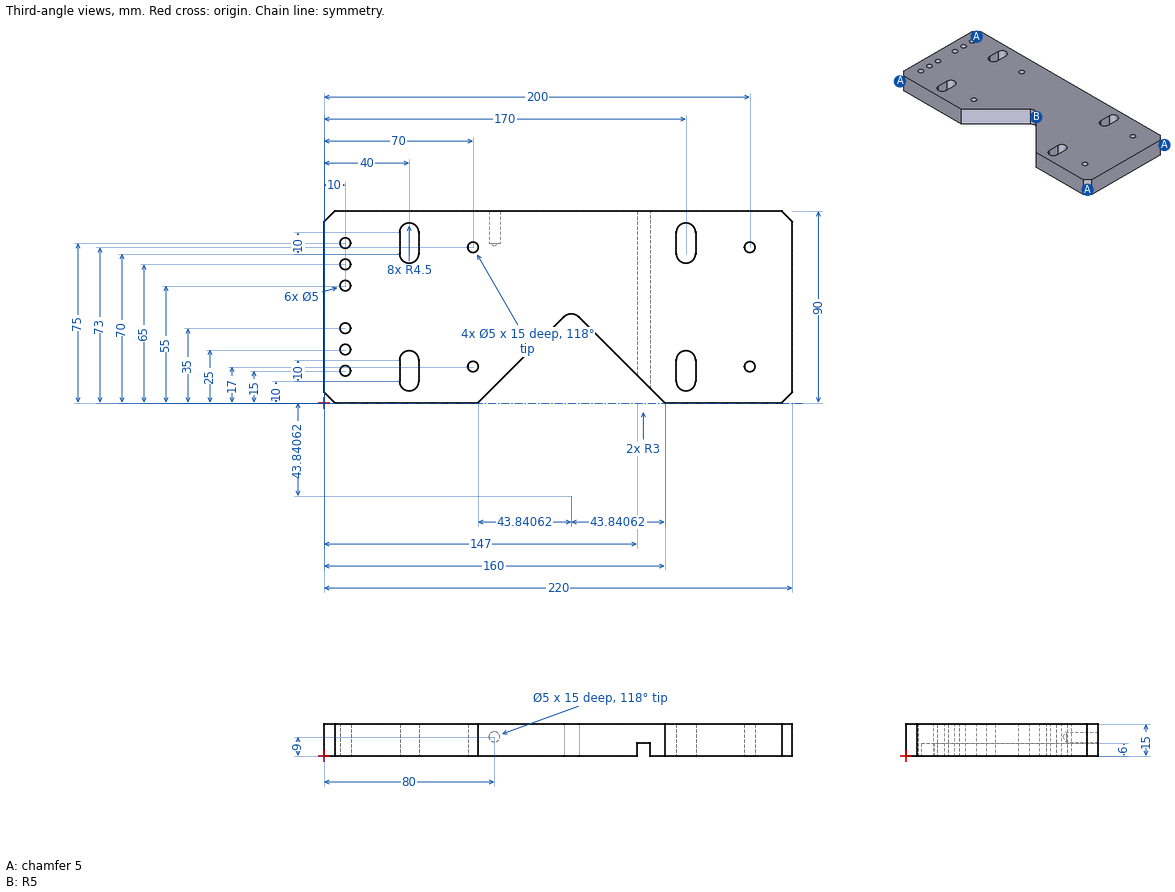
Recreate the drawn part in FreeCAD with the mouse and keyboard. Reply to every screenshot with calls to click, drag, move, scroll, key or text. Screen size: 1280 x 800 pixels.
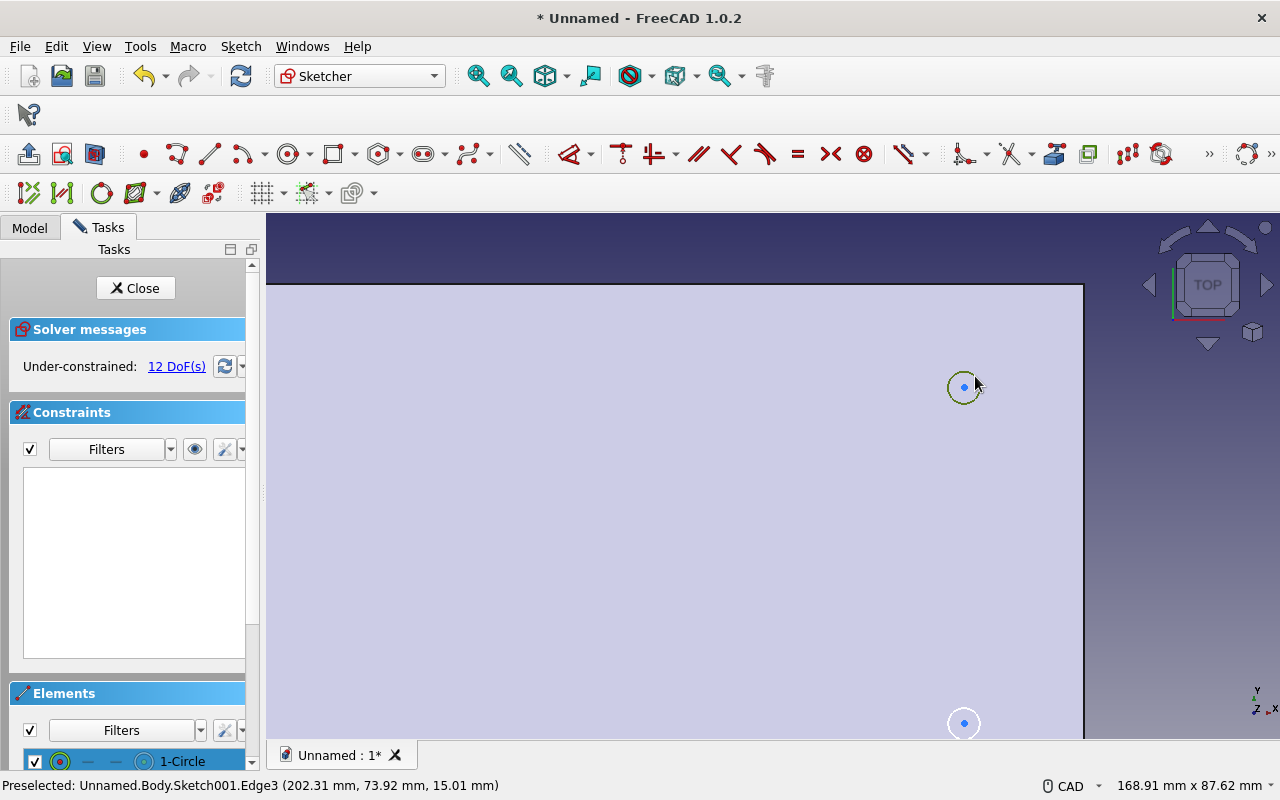
click(964, 708)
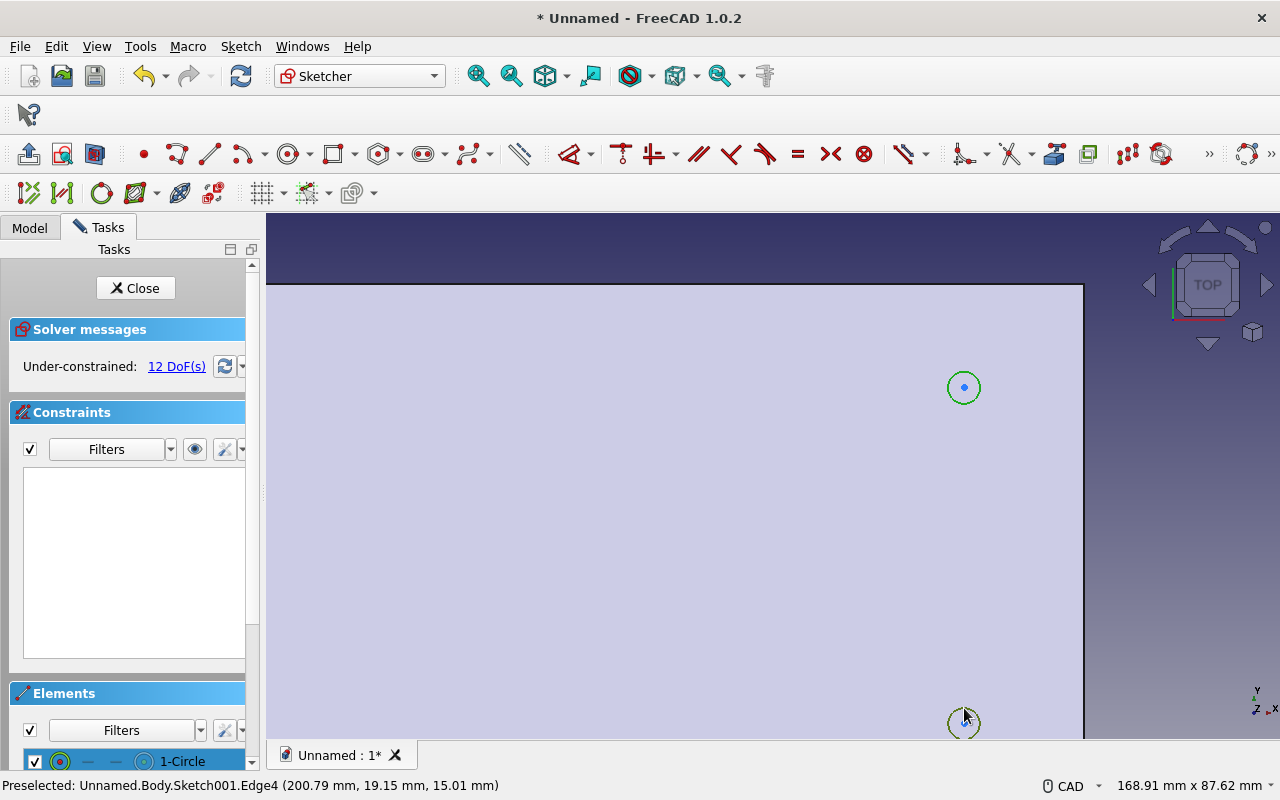
click(798, 154)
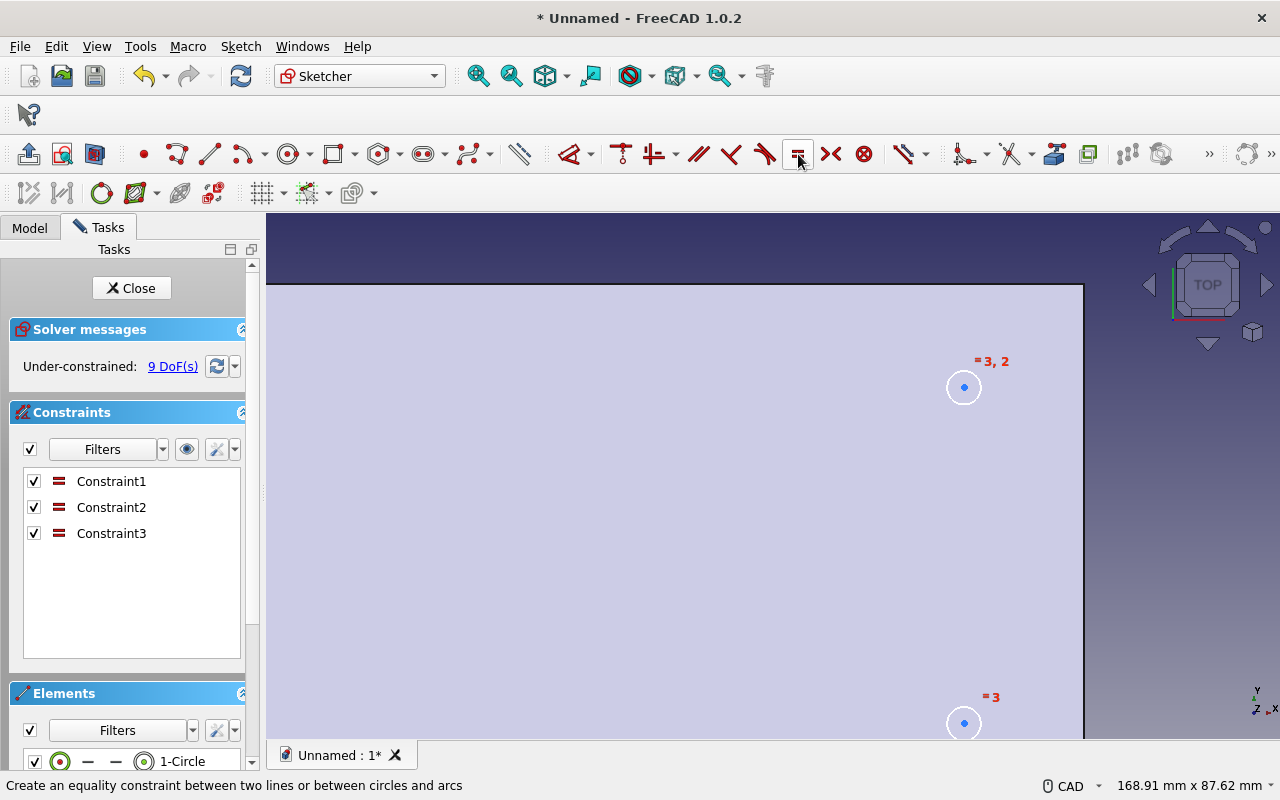
click(568, 154)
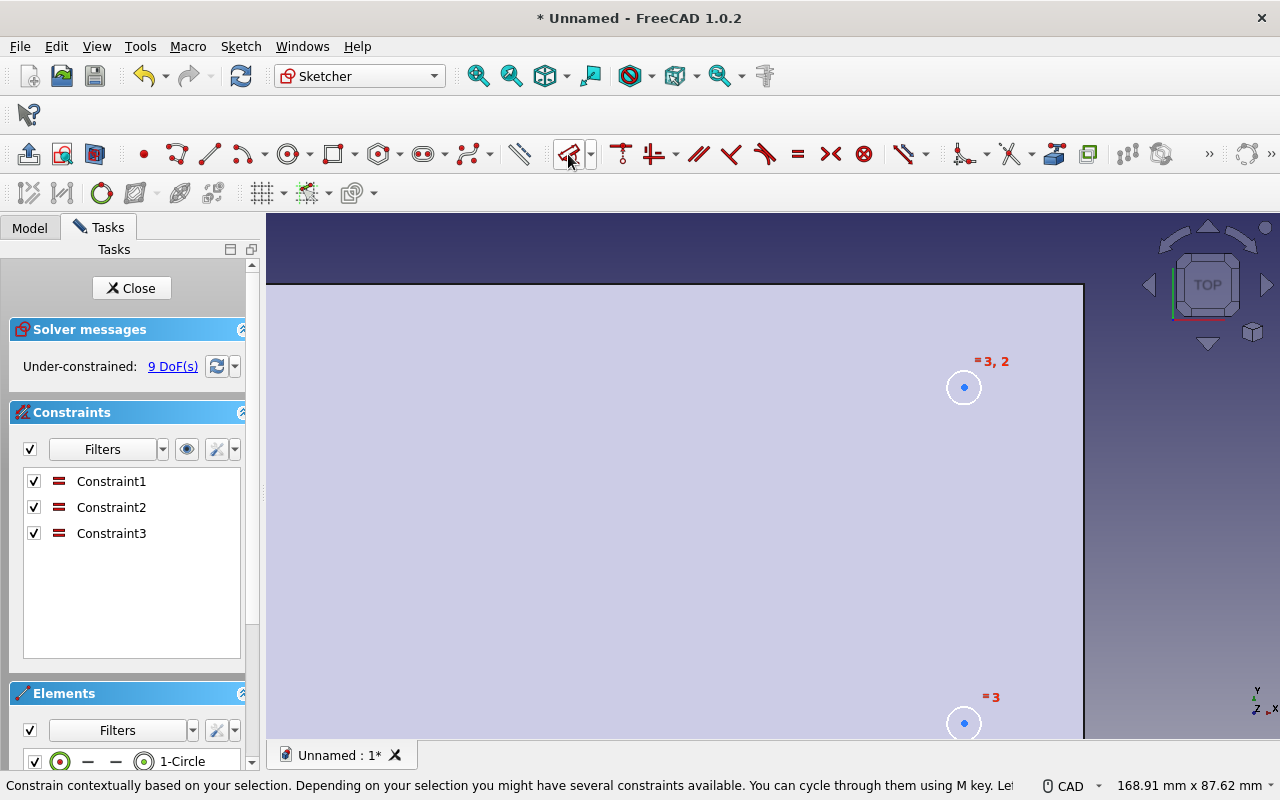
scroll(976, 377, down, 4)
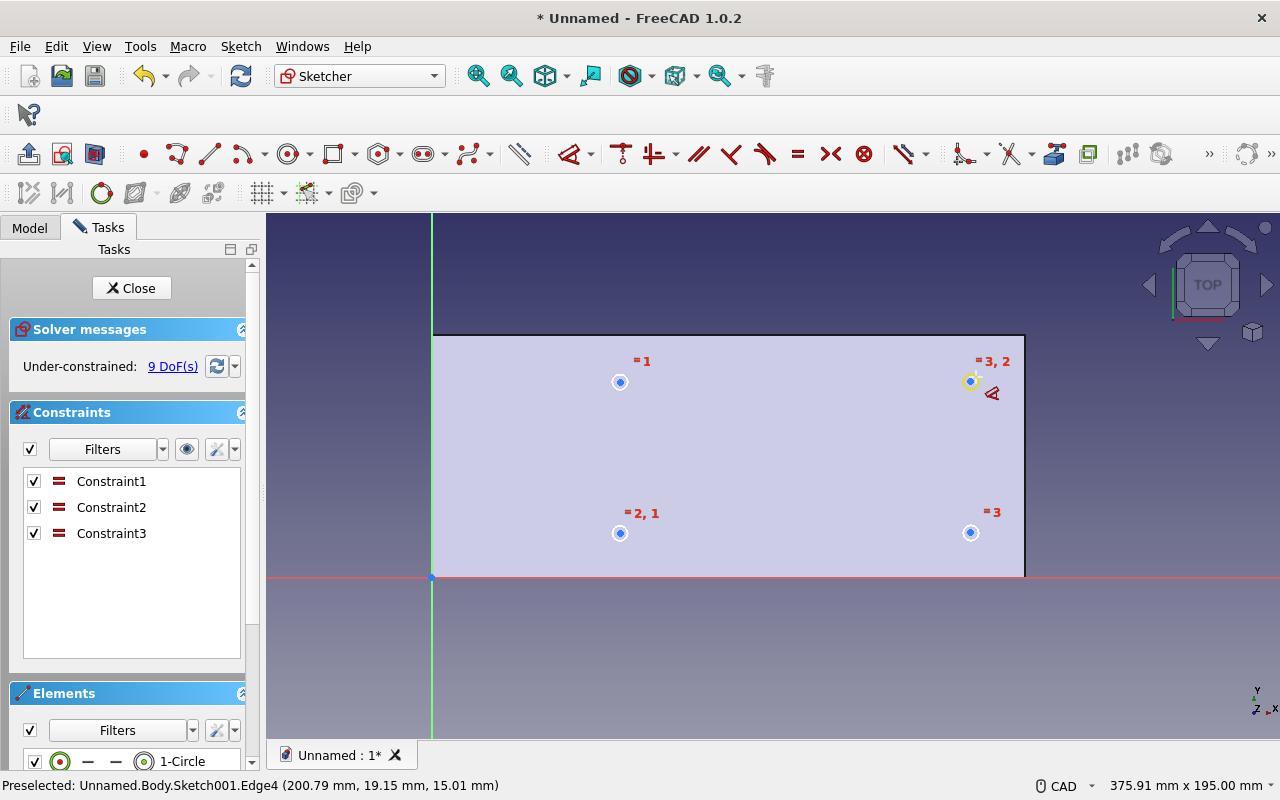
scroll(625, 377, up, 6)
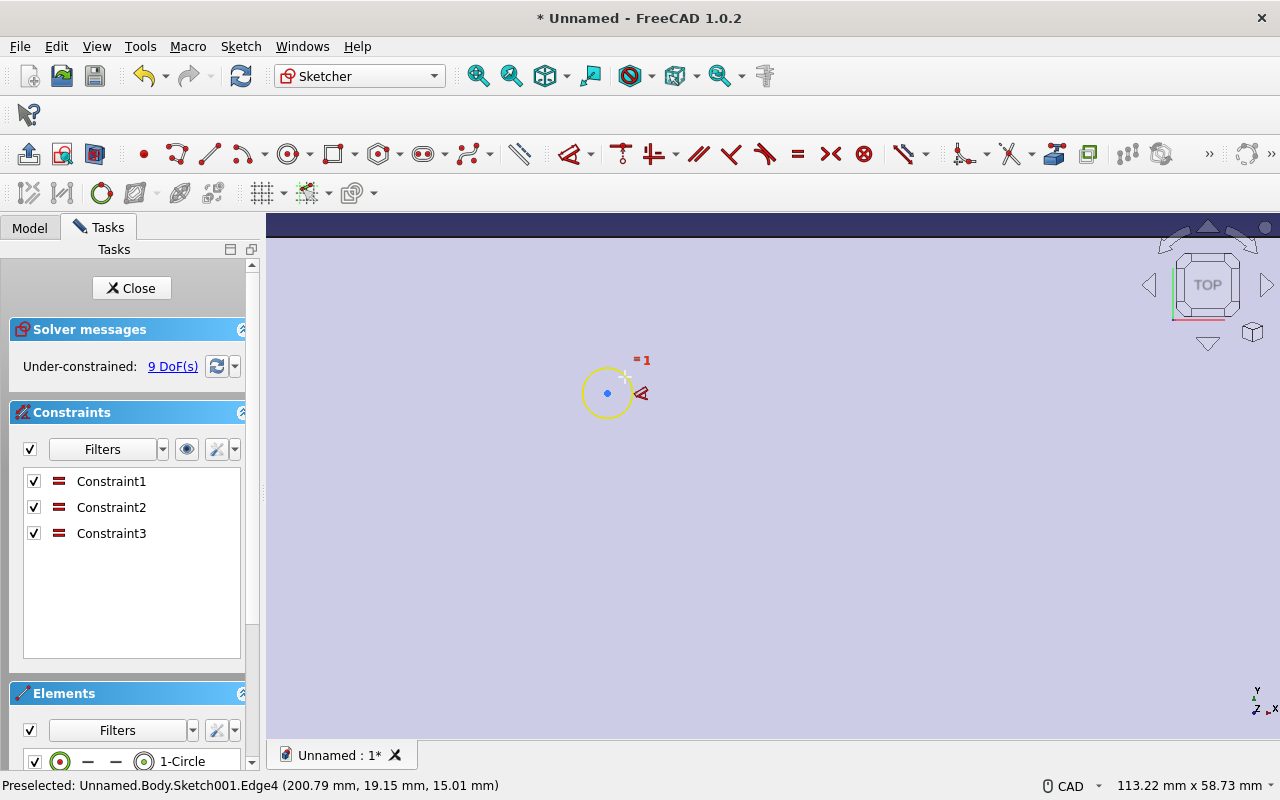
click(625, 376)
click(648, 353)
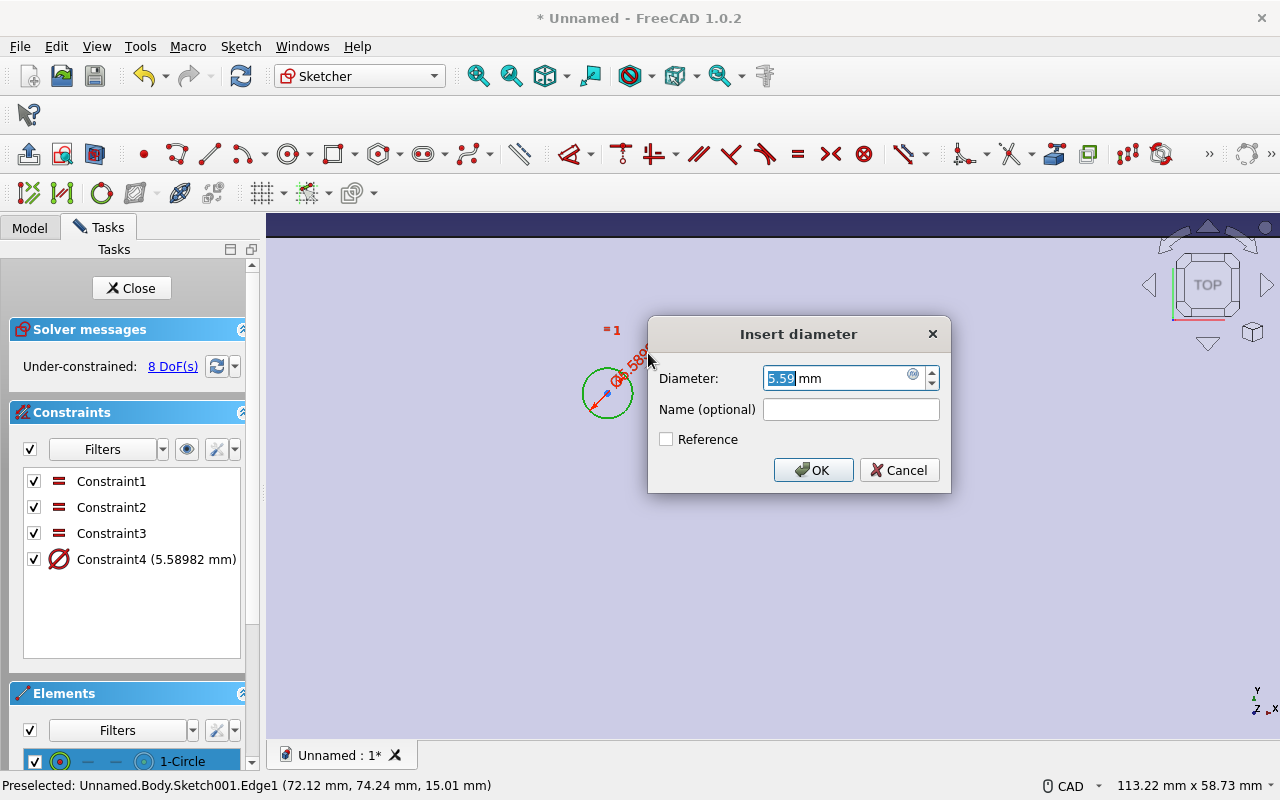
text(5)
key(Return)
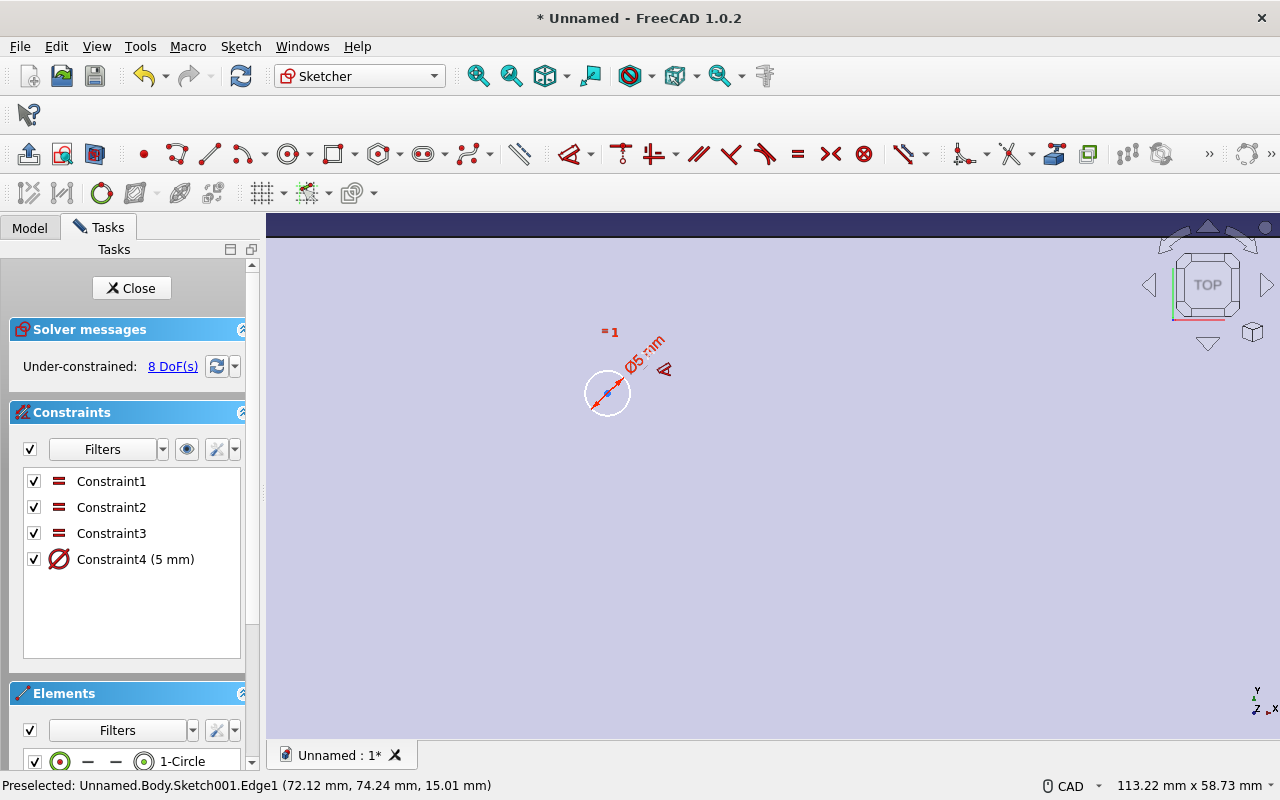
scroll(625, 377, down, 6)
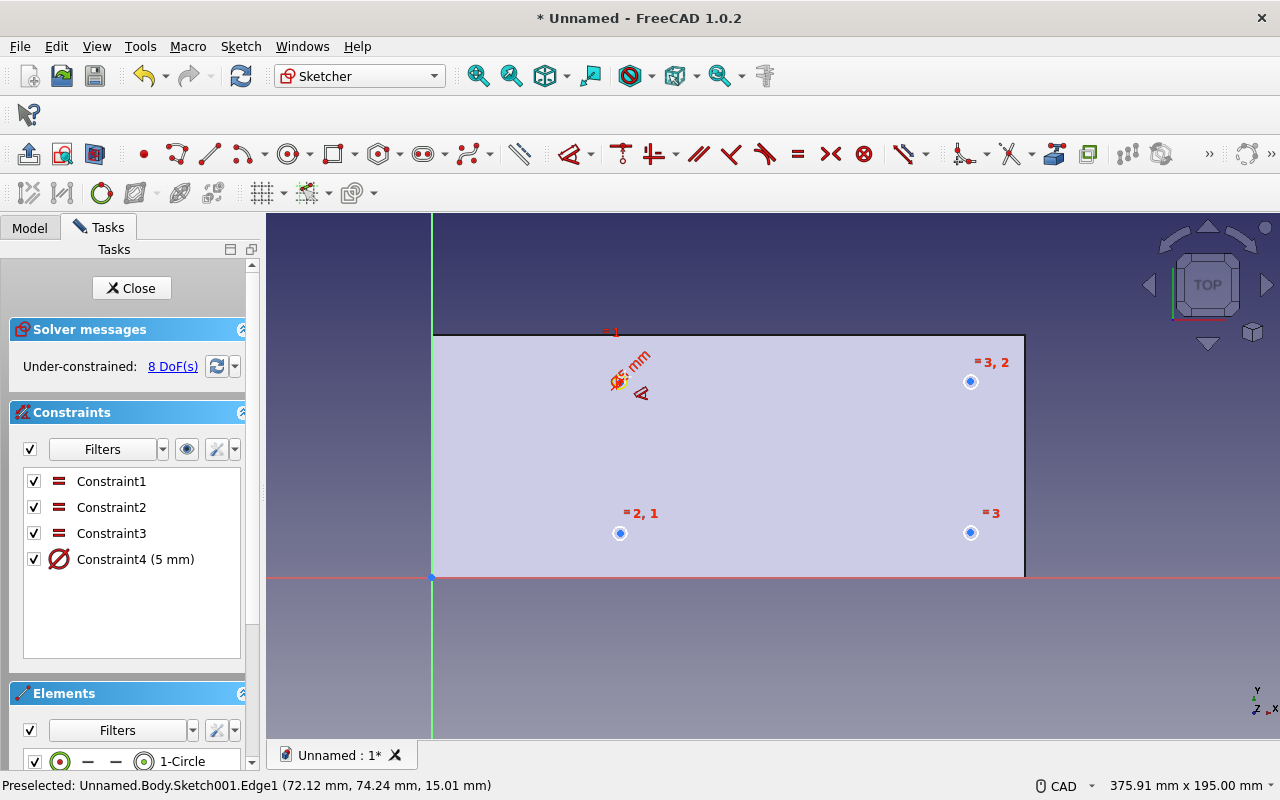
click(620, 382)
click(526, 612)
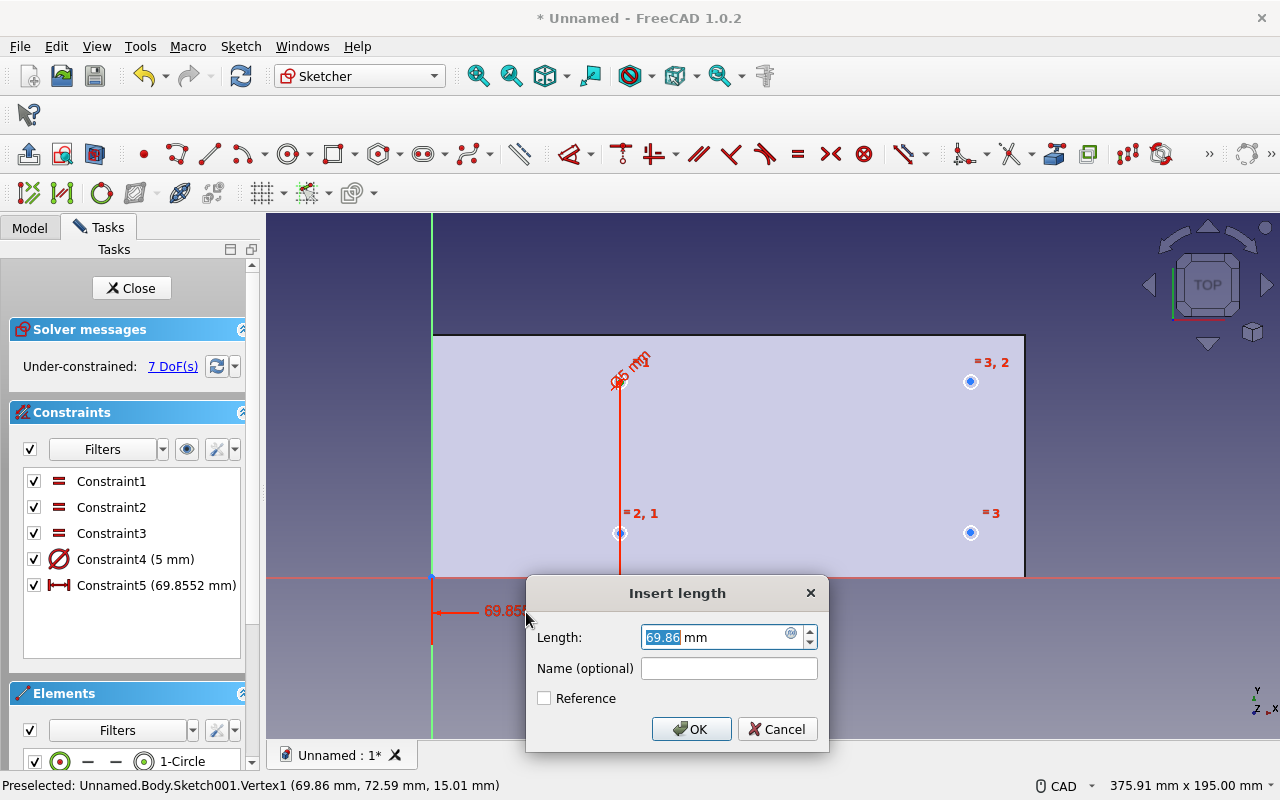
text(70)
key(Return)